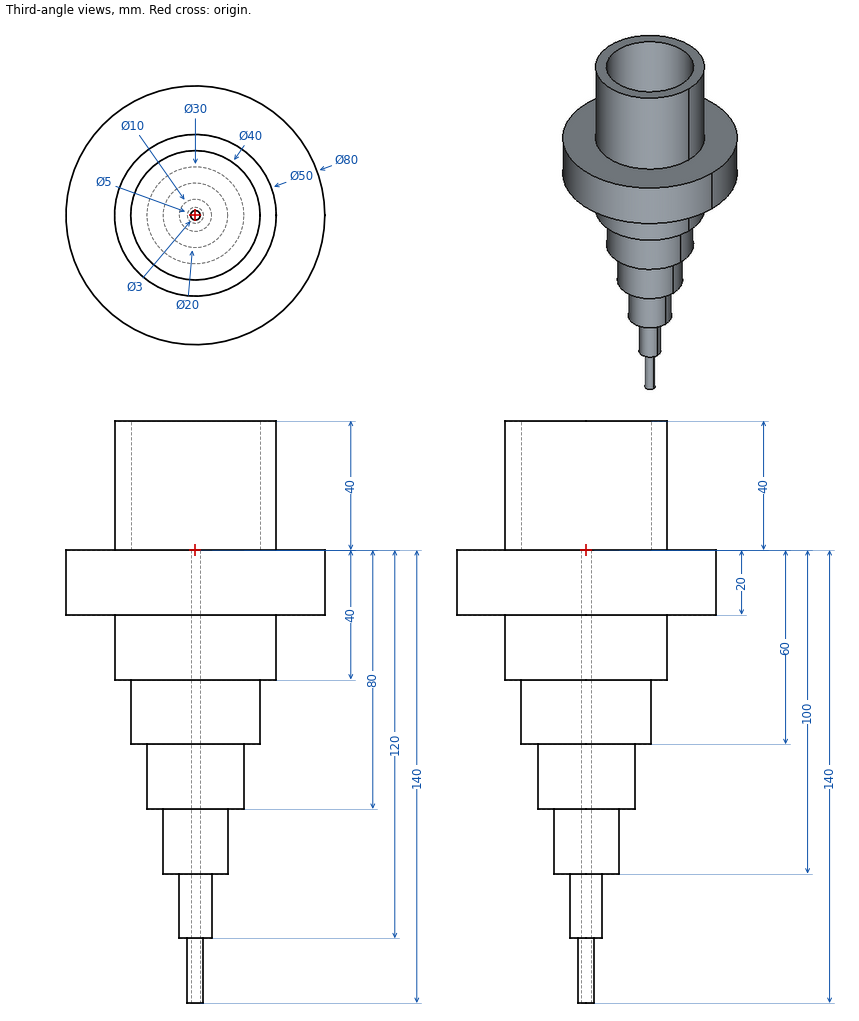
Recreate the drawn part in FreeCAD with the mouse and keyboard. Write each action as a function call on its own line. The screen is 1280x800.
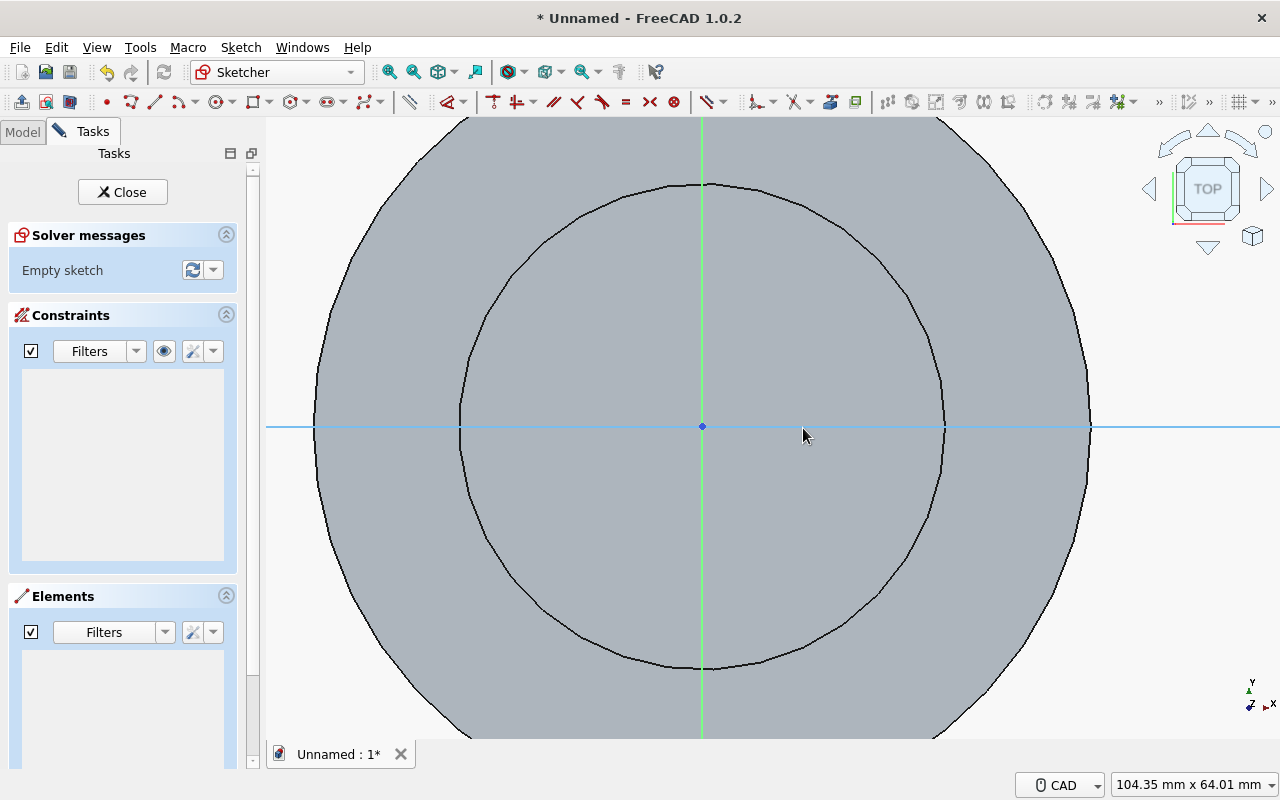
key(g)
key(c)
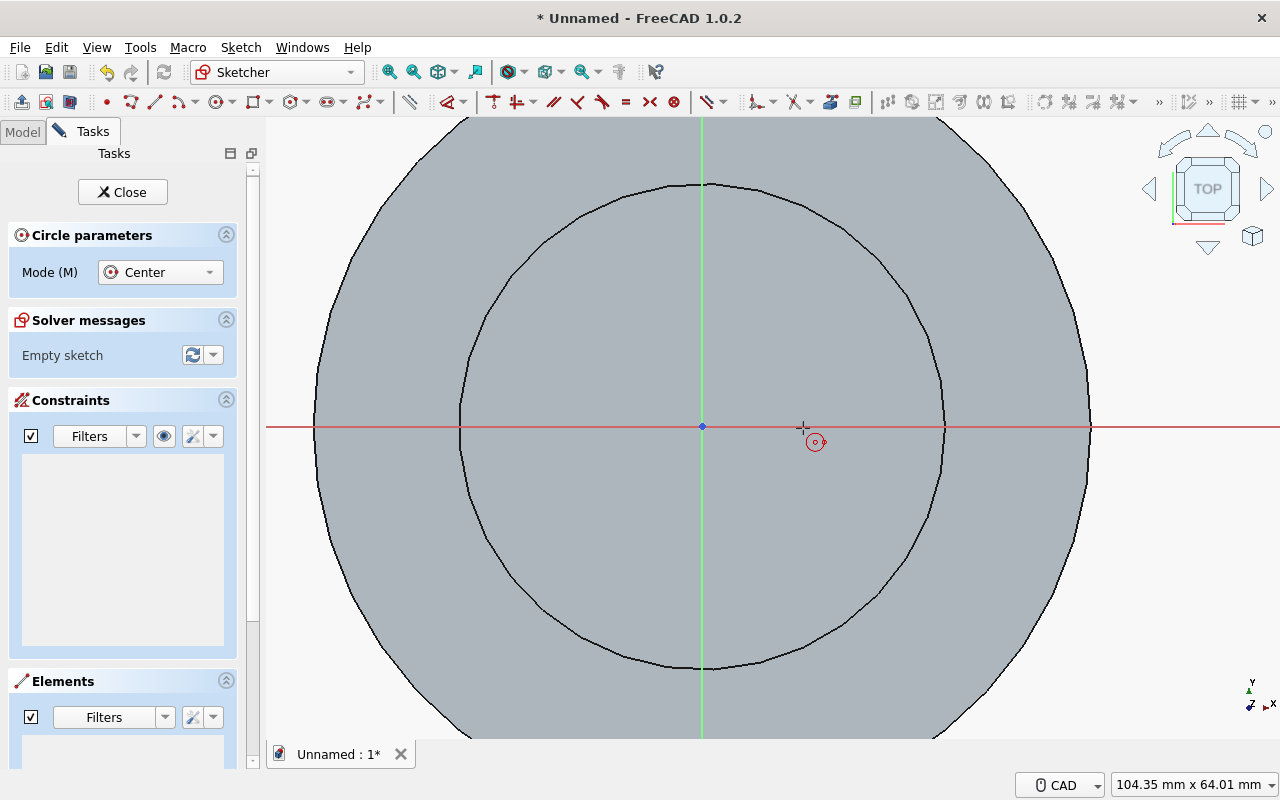
click(702, 427)
move(840, 289)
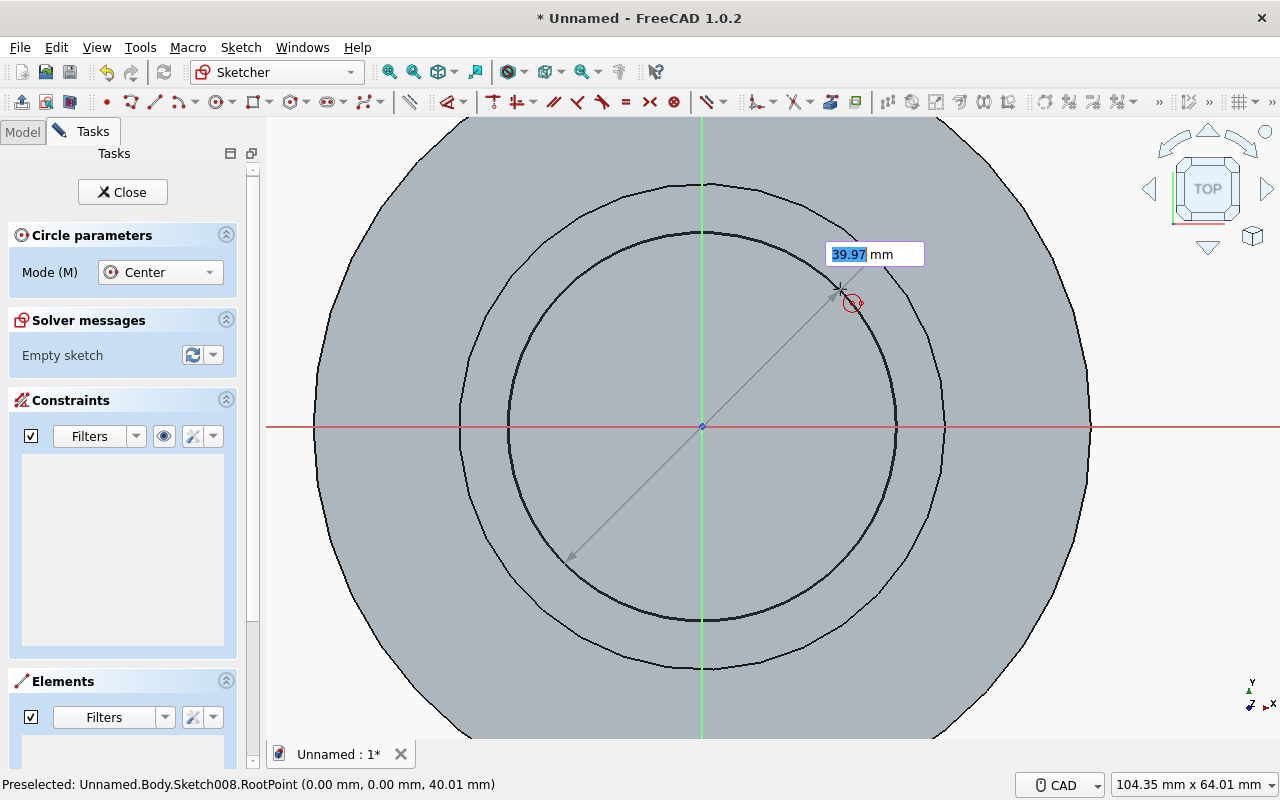
text(40)
key(Return)
key(Escape)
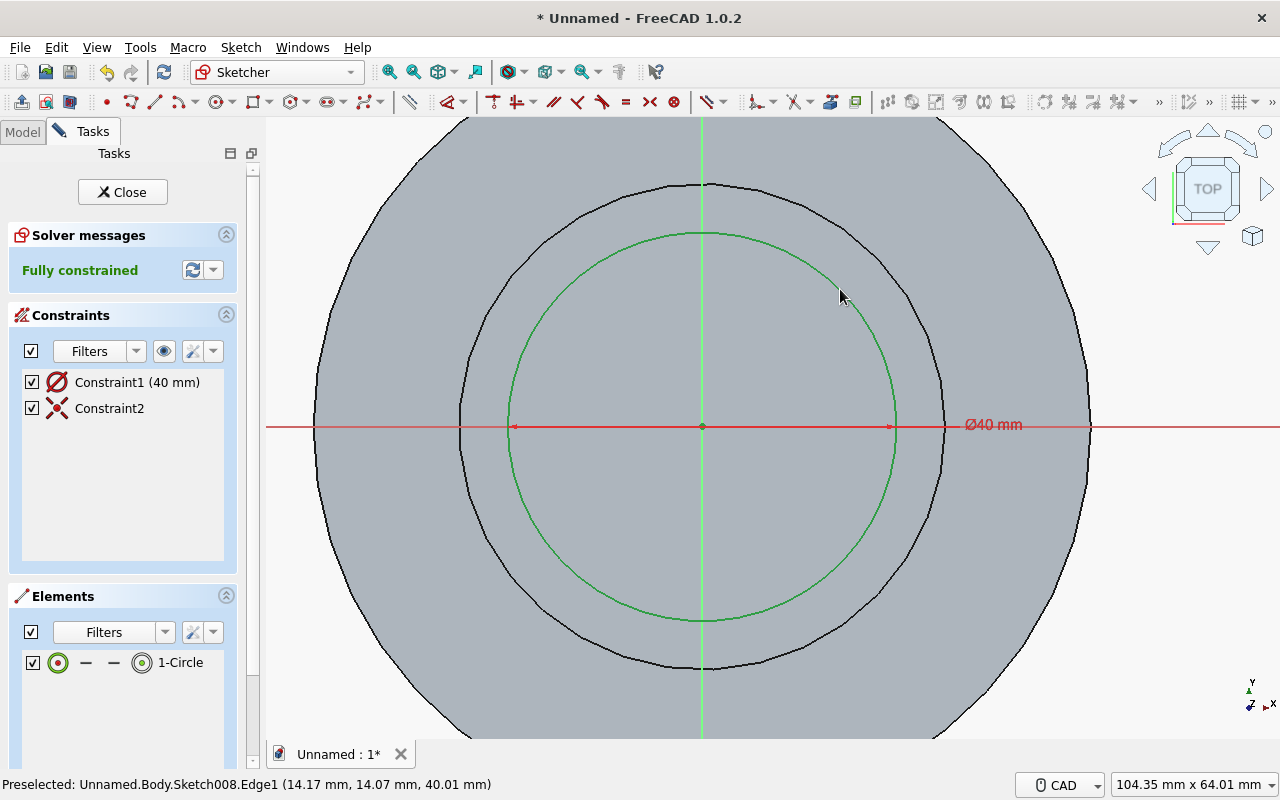
click(123, 192)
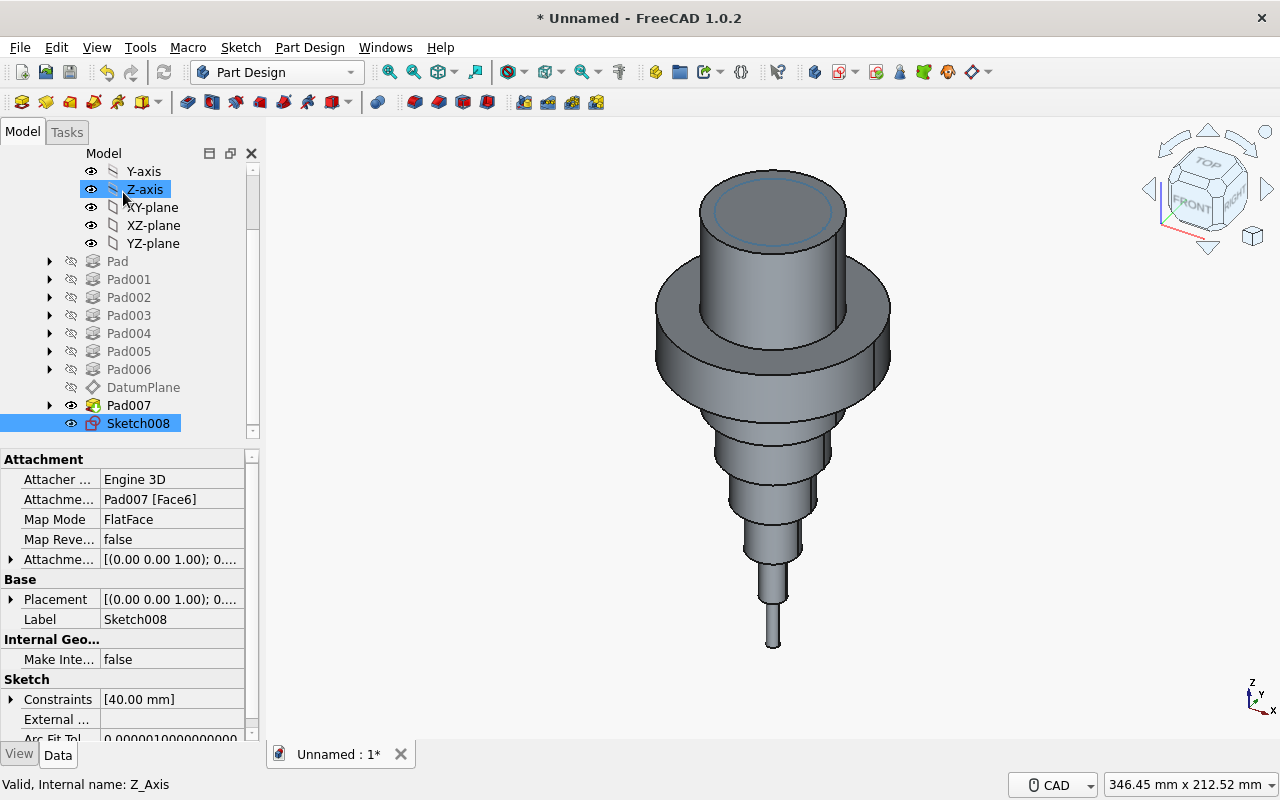
click(188, 102)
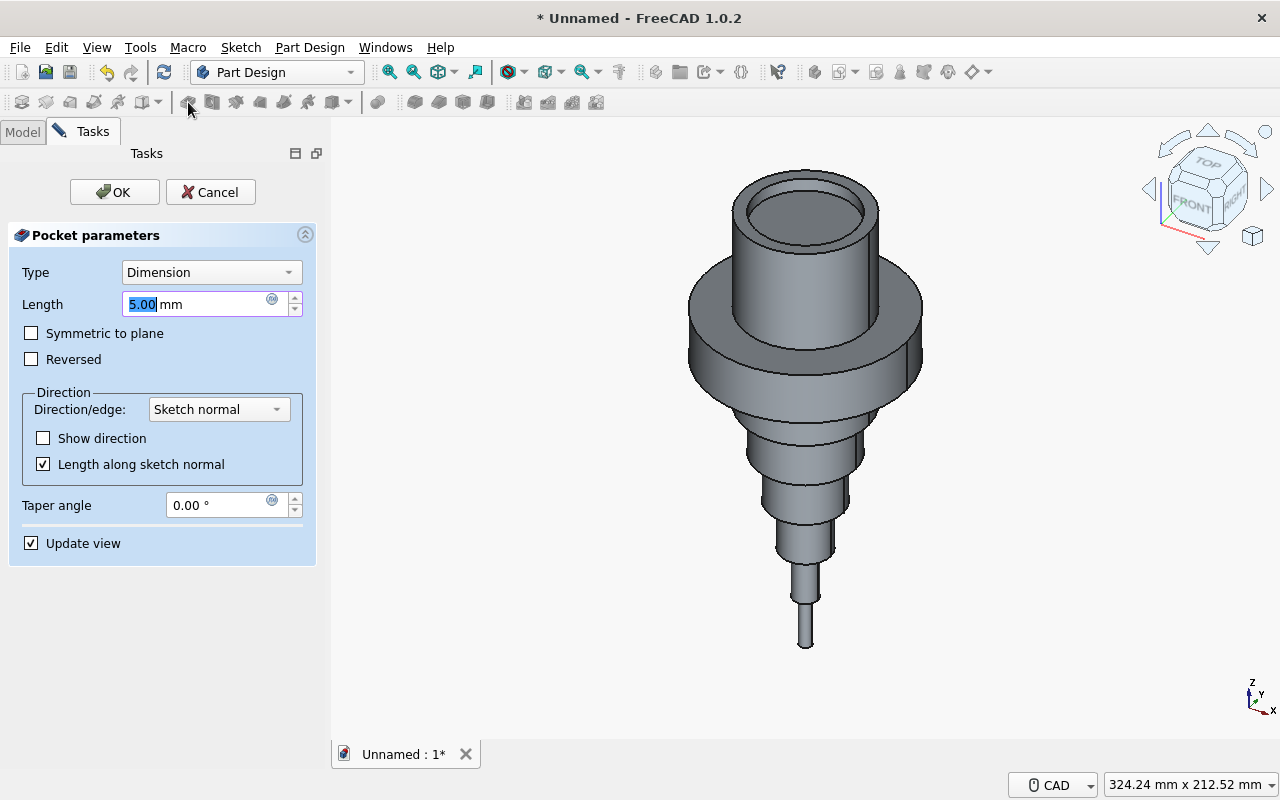
text(40)
key(Tab)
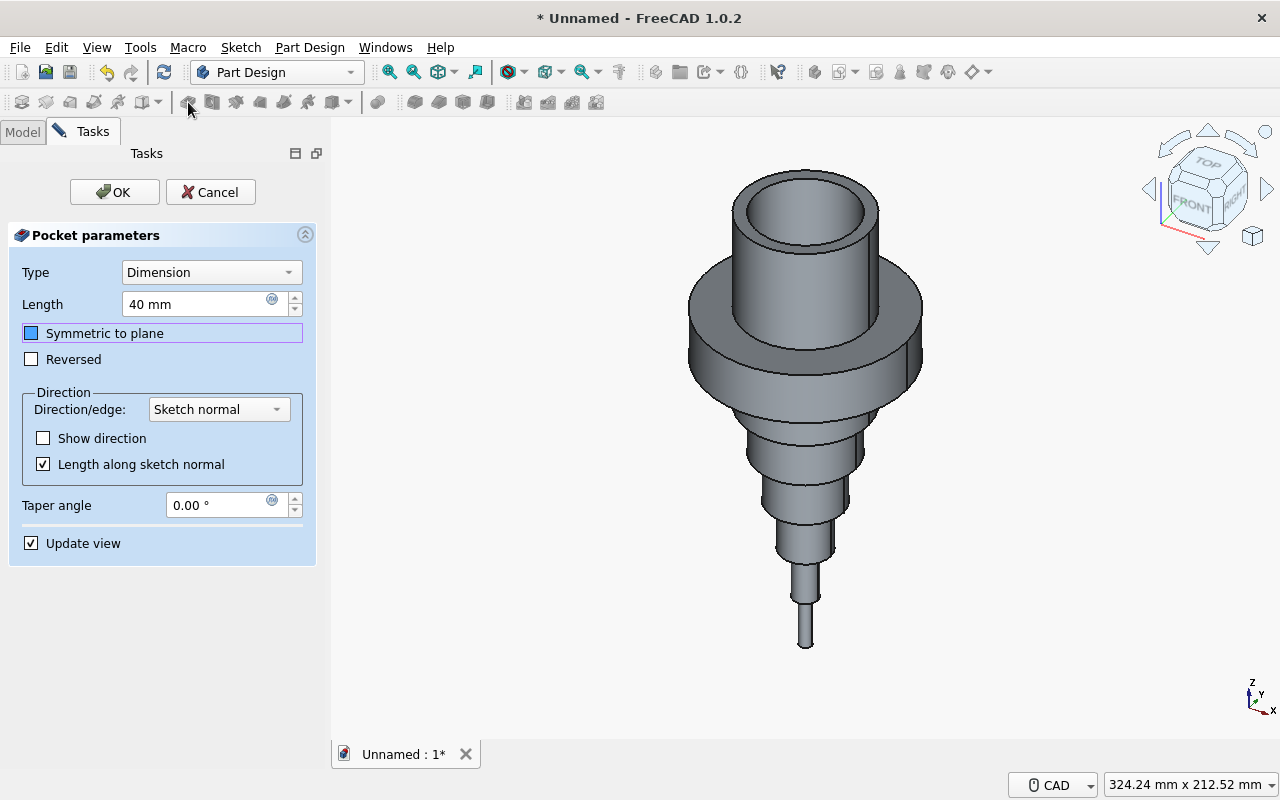
click(115, 192)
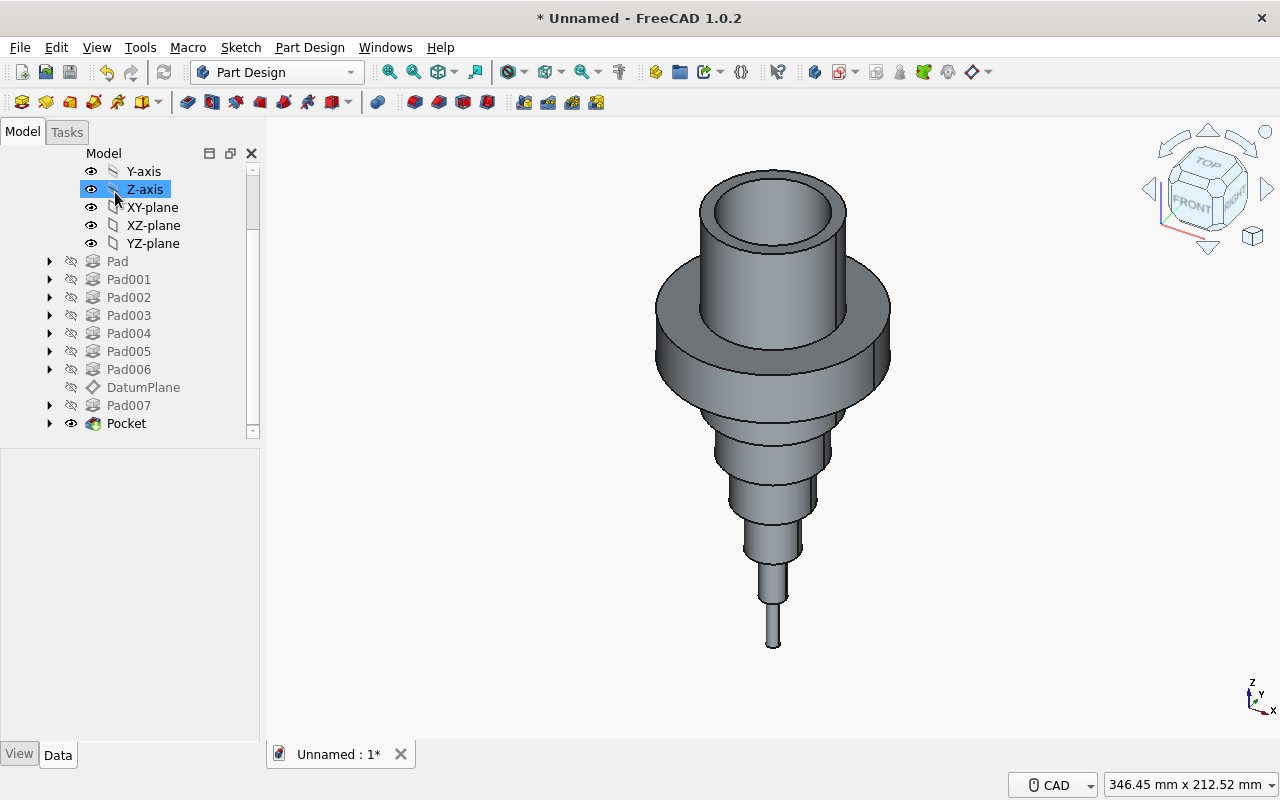
click(840, 72)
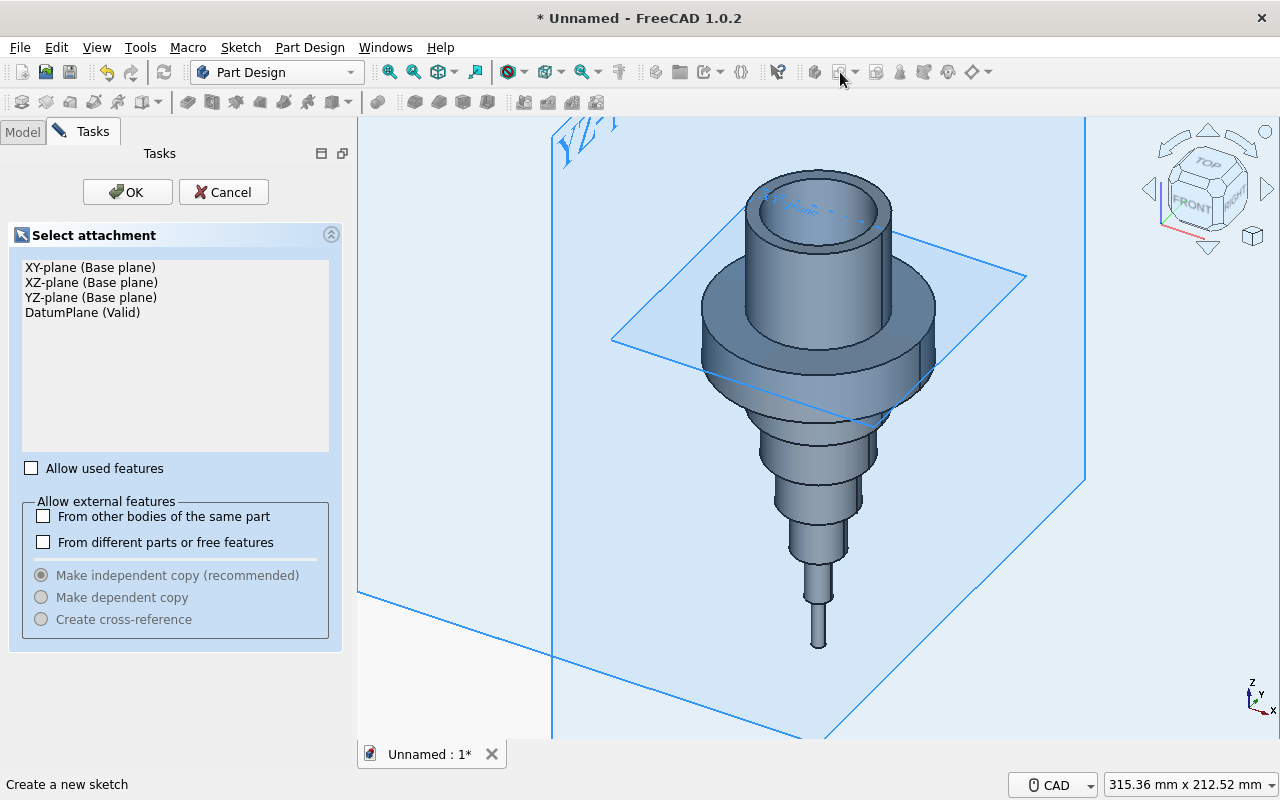
click(82, 268)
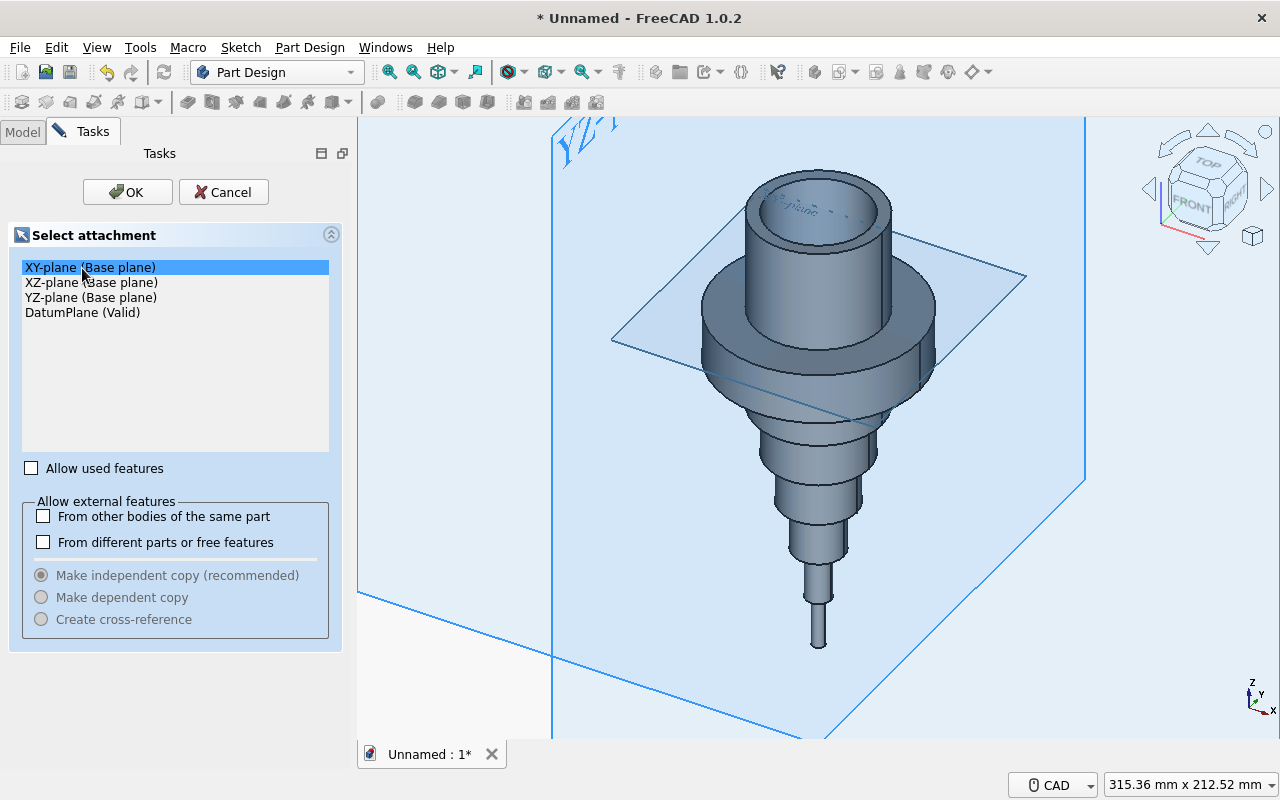
click(128, 192)